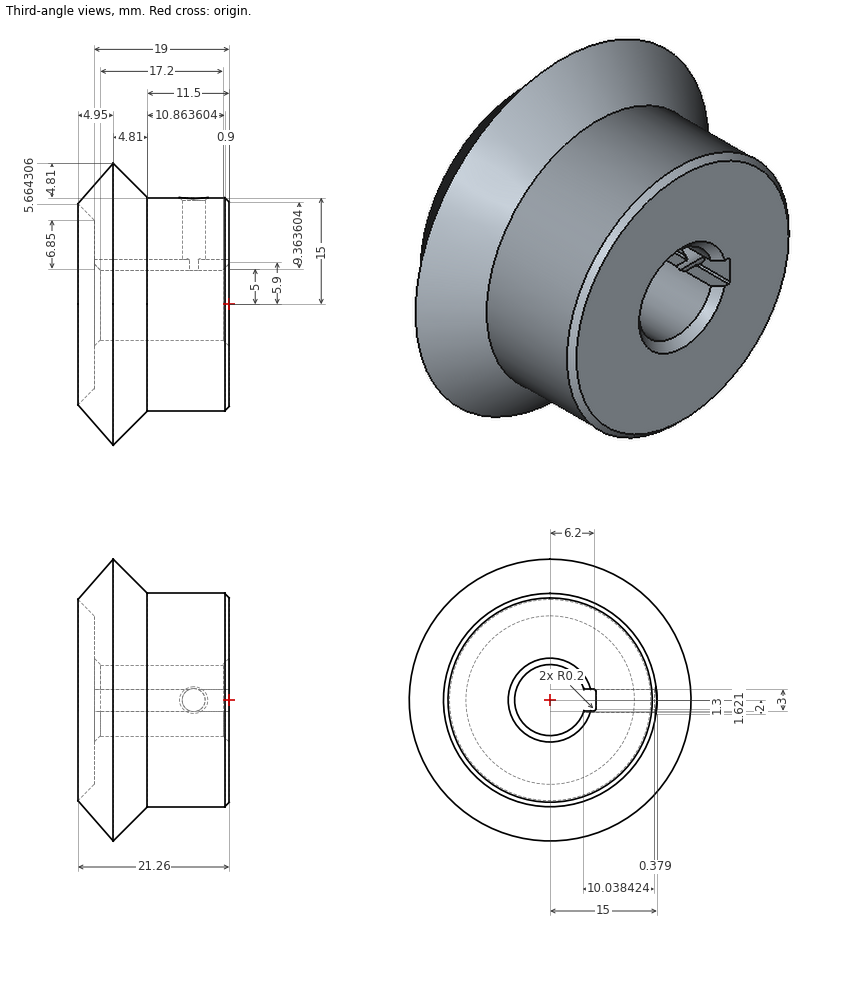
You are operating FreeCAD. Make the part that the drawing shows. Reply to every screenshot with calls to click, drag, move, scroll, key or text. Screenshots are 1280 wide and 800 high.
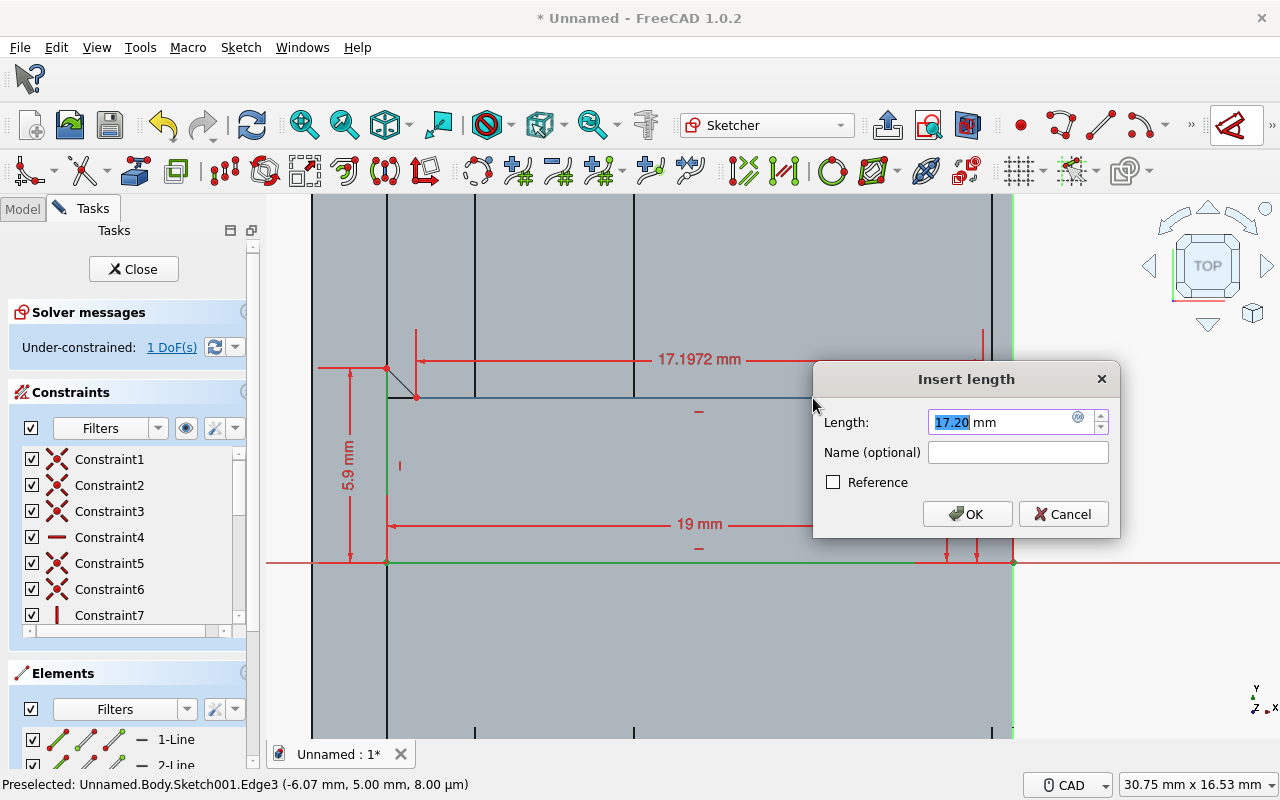
text(17.2)
key(Return)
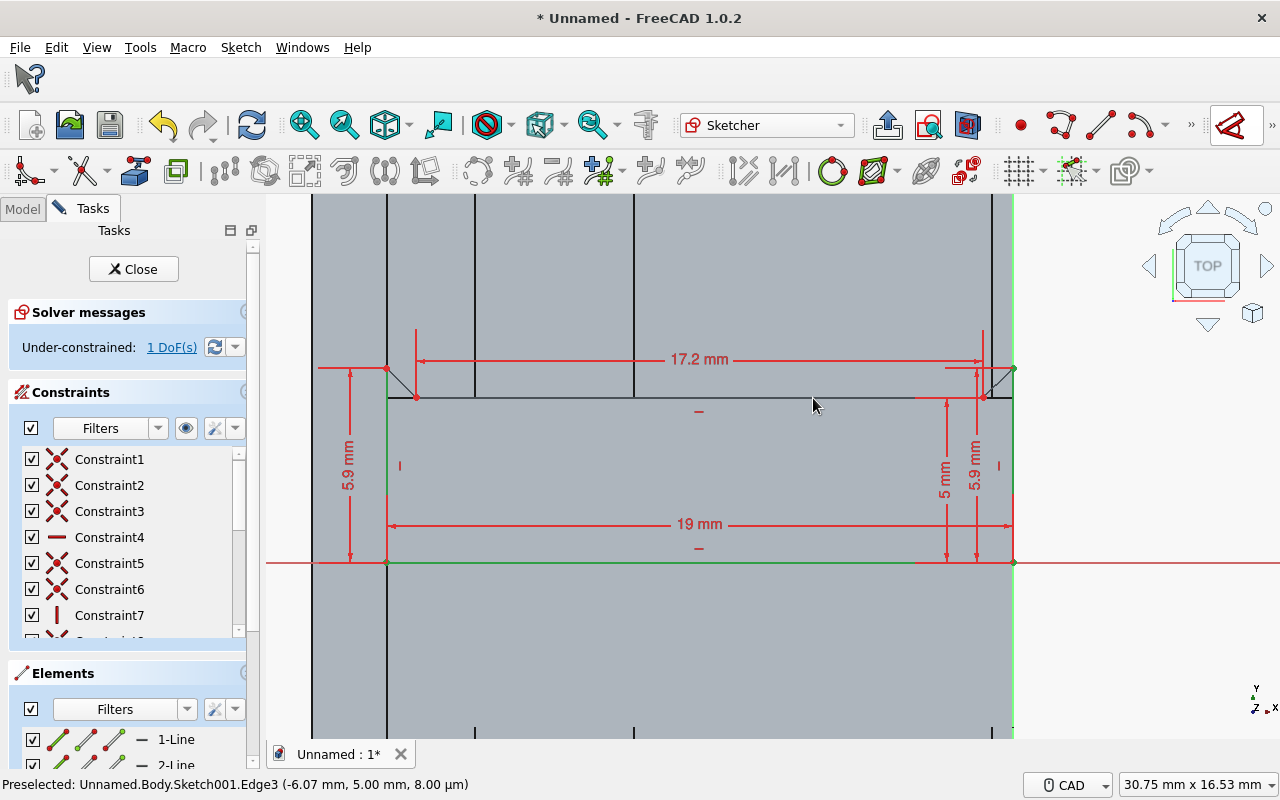
scroll(983, 398, up, 2)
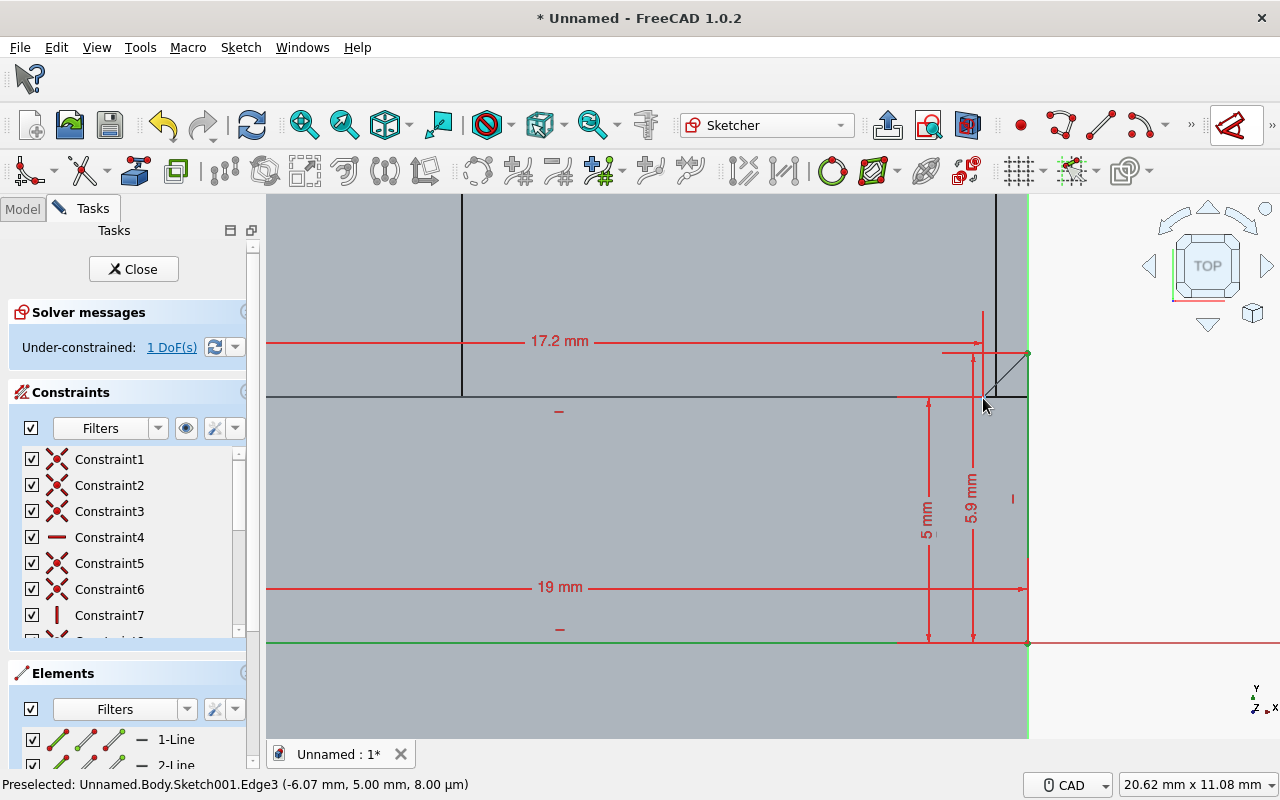
click(983, 397)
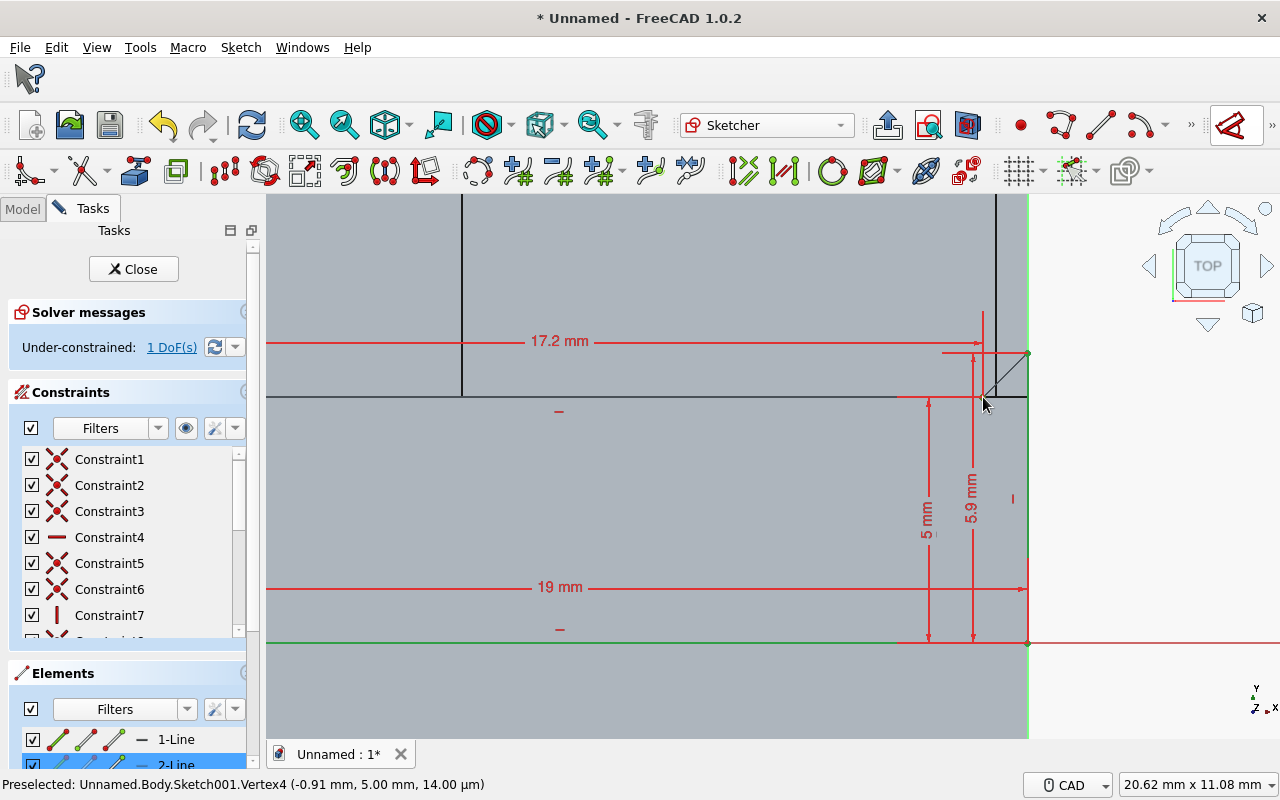
click(1258, 126)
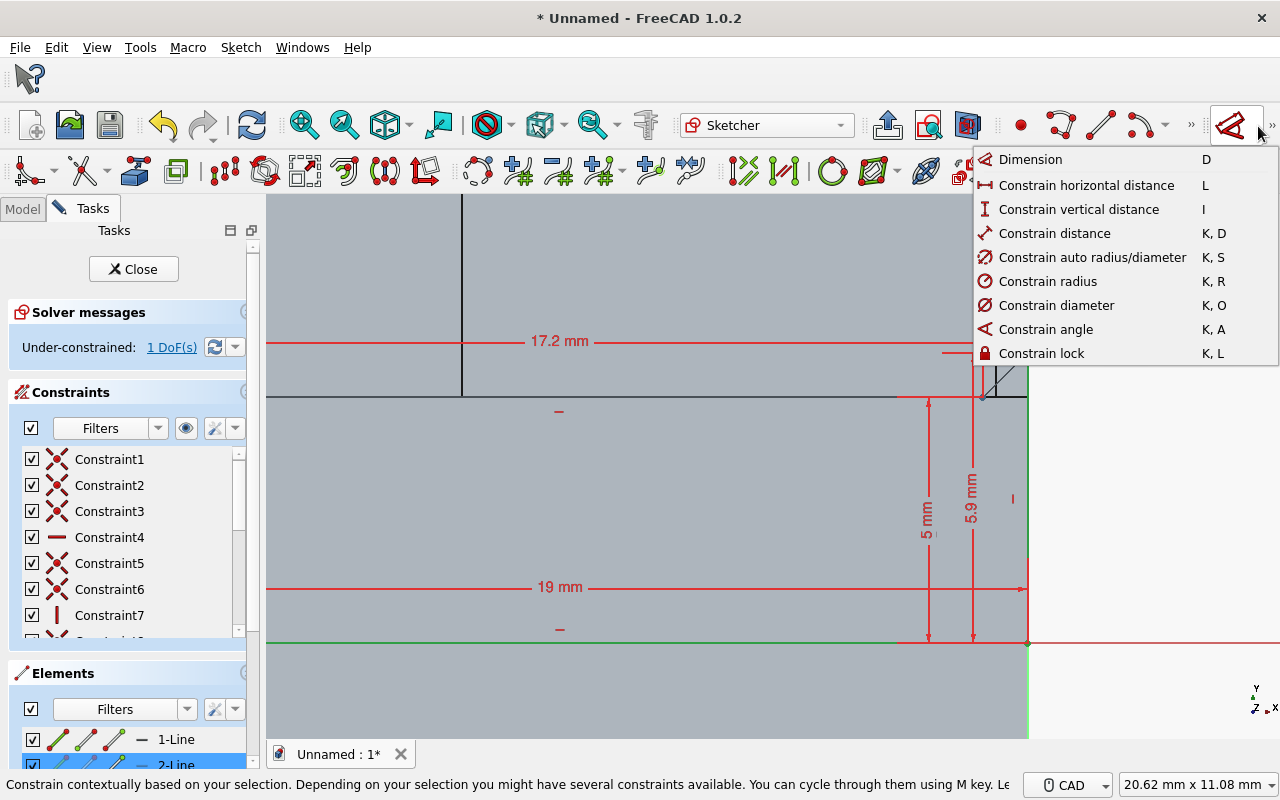
click(1126, 185)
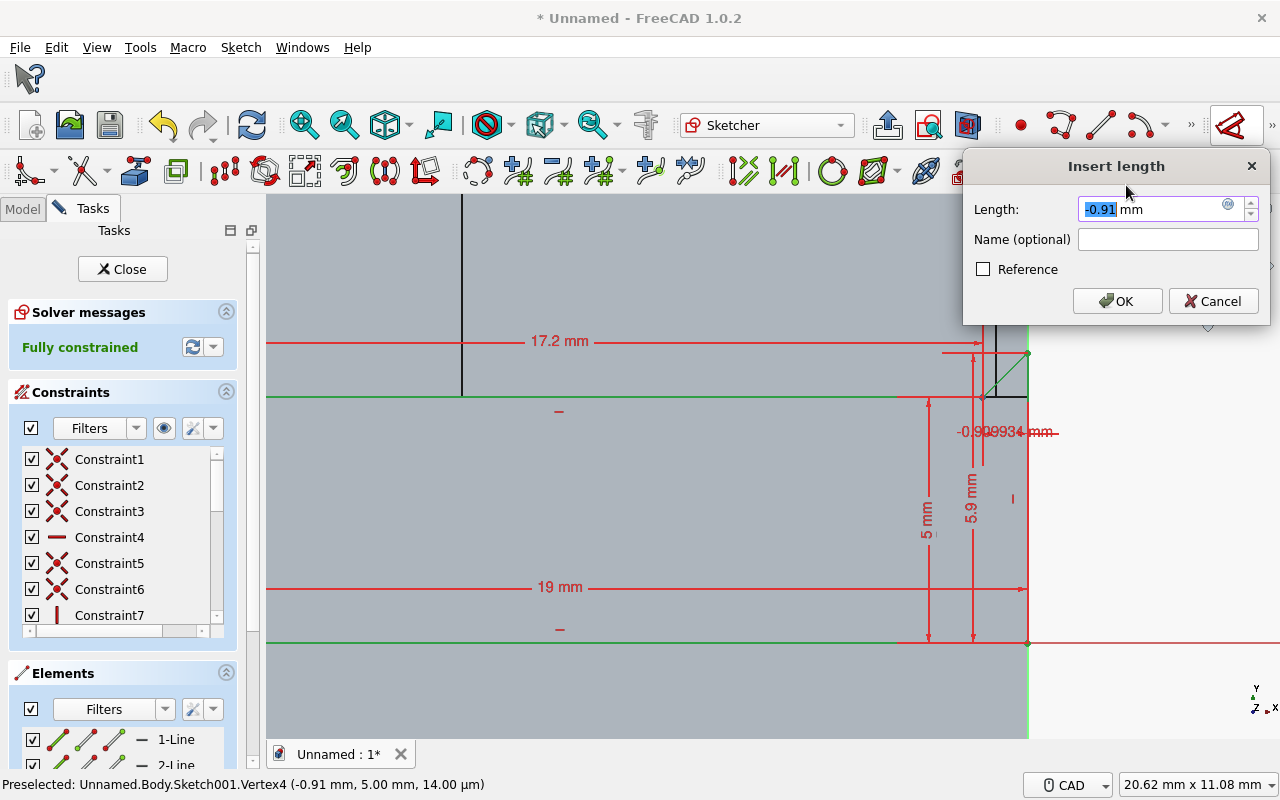
text(-0.9)
key(Return)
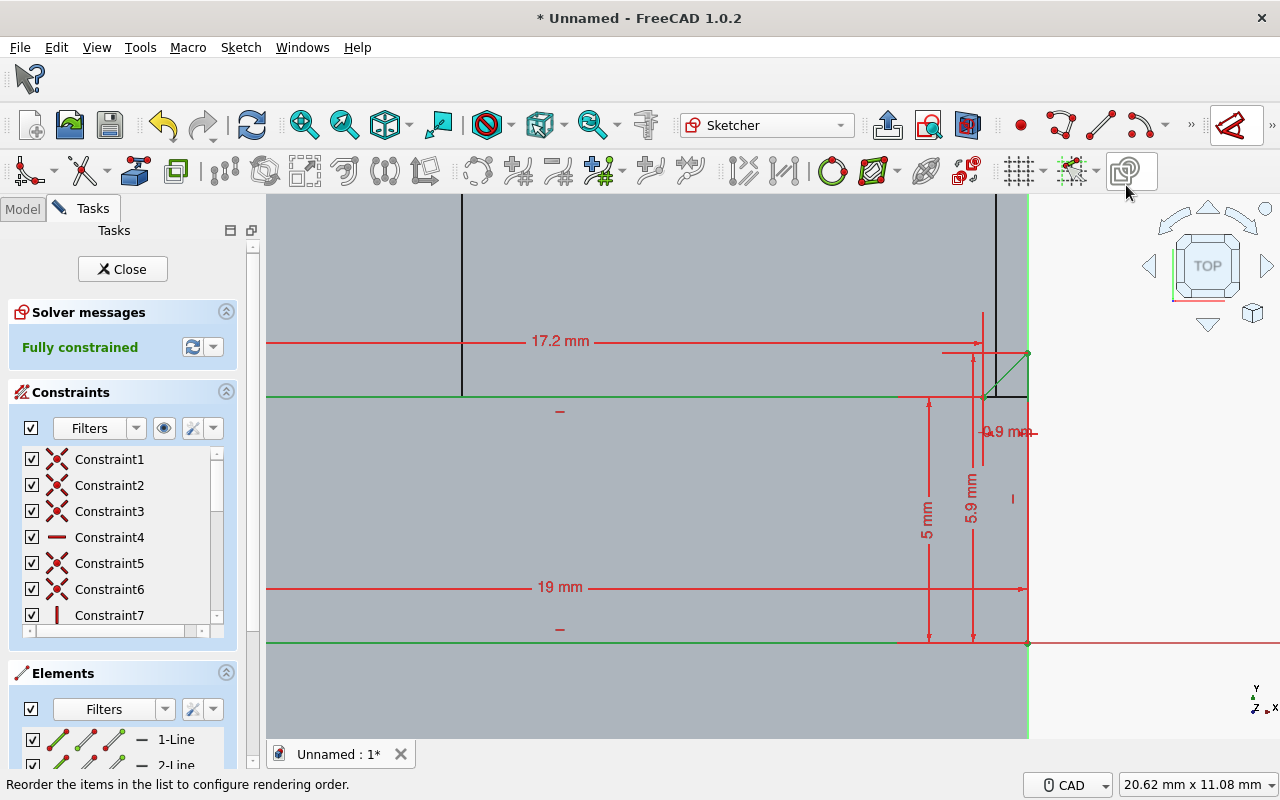
click(123, 269)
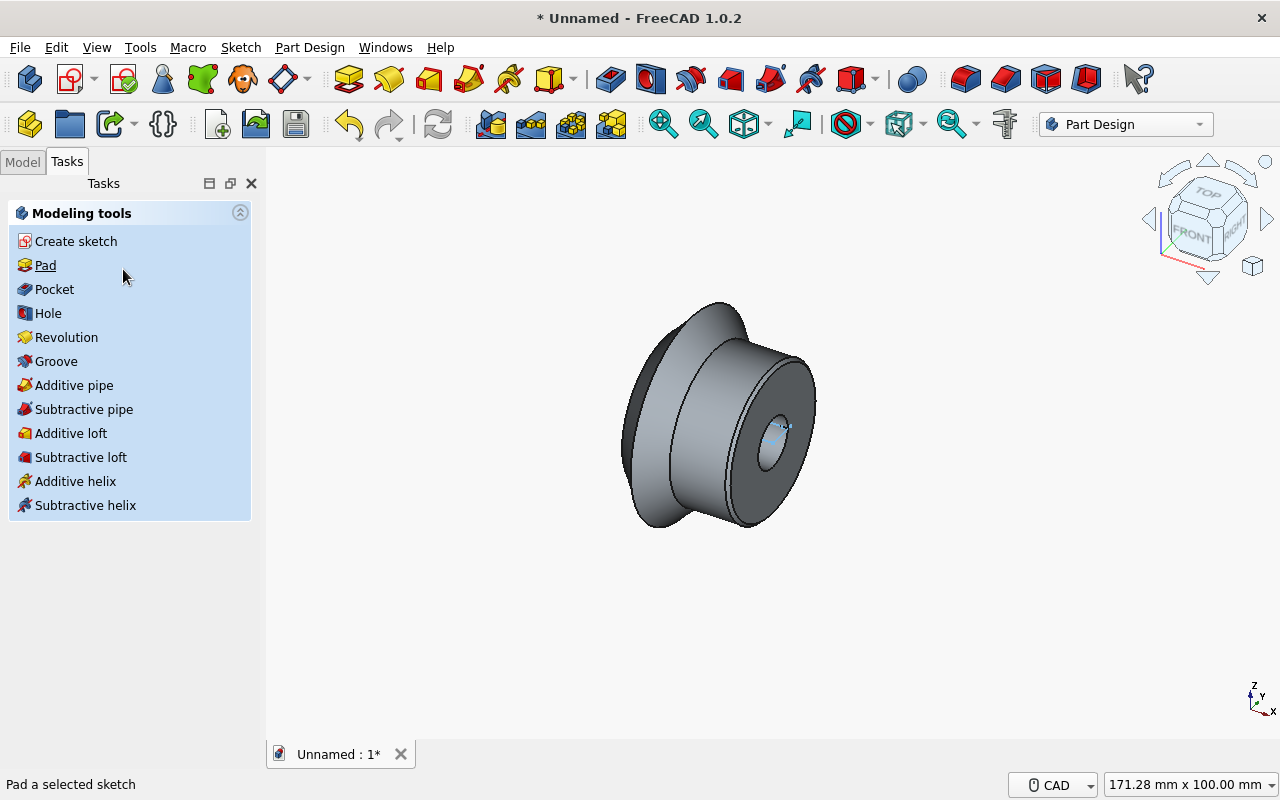
click(692, 80)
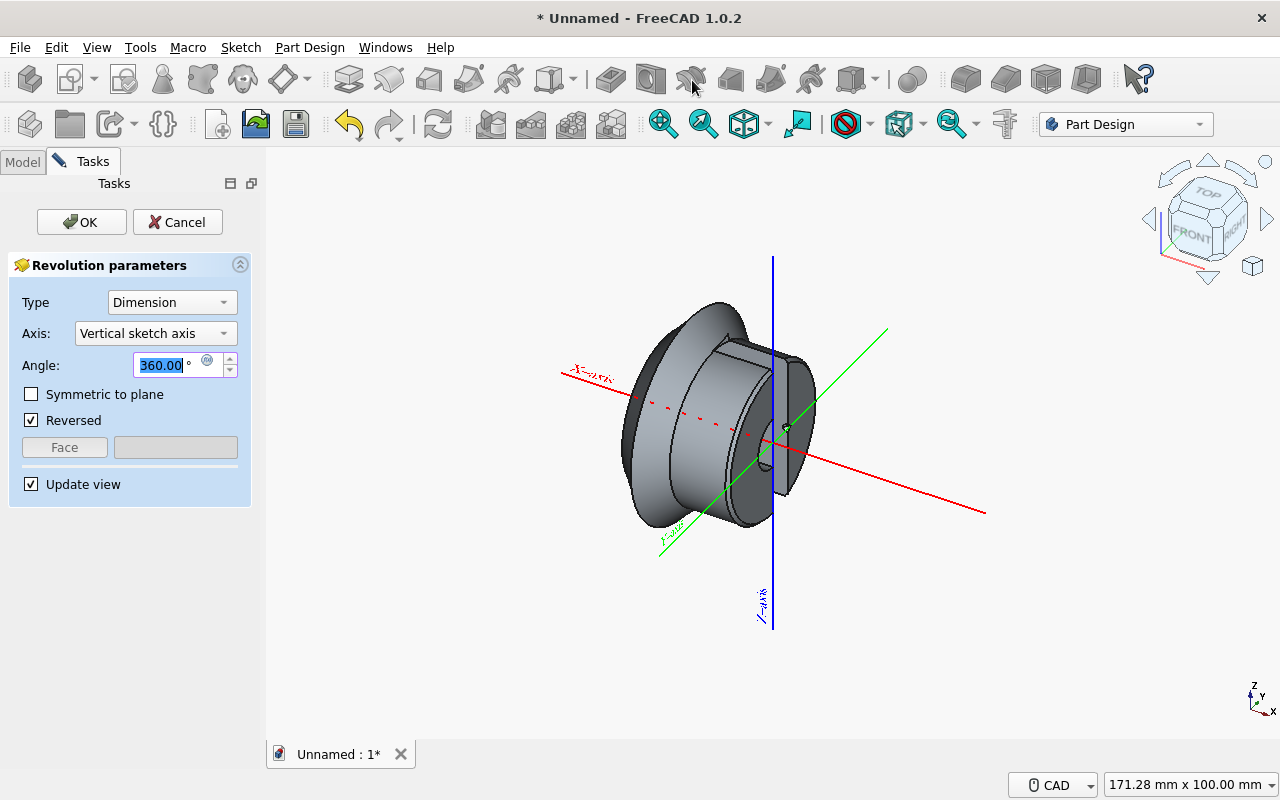
click(156, 334)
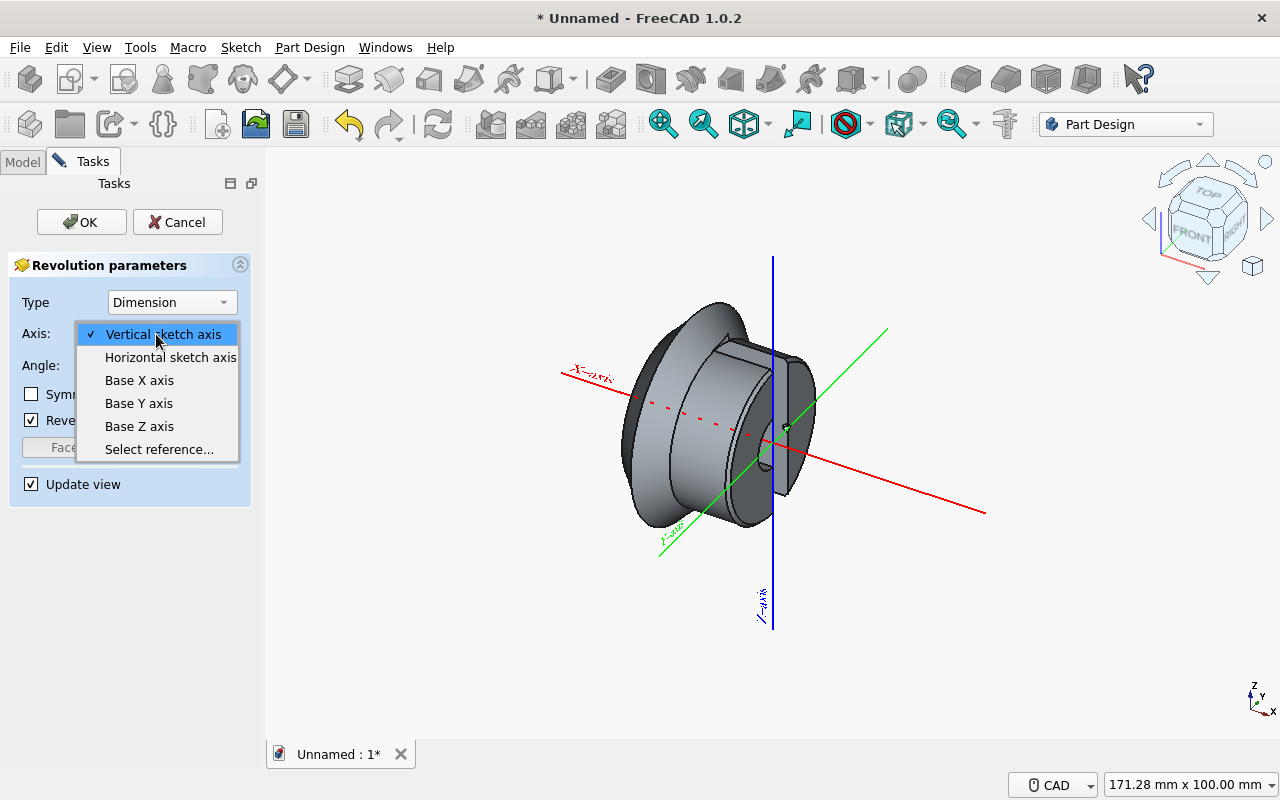
click(156, 358)